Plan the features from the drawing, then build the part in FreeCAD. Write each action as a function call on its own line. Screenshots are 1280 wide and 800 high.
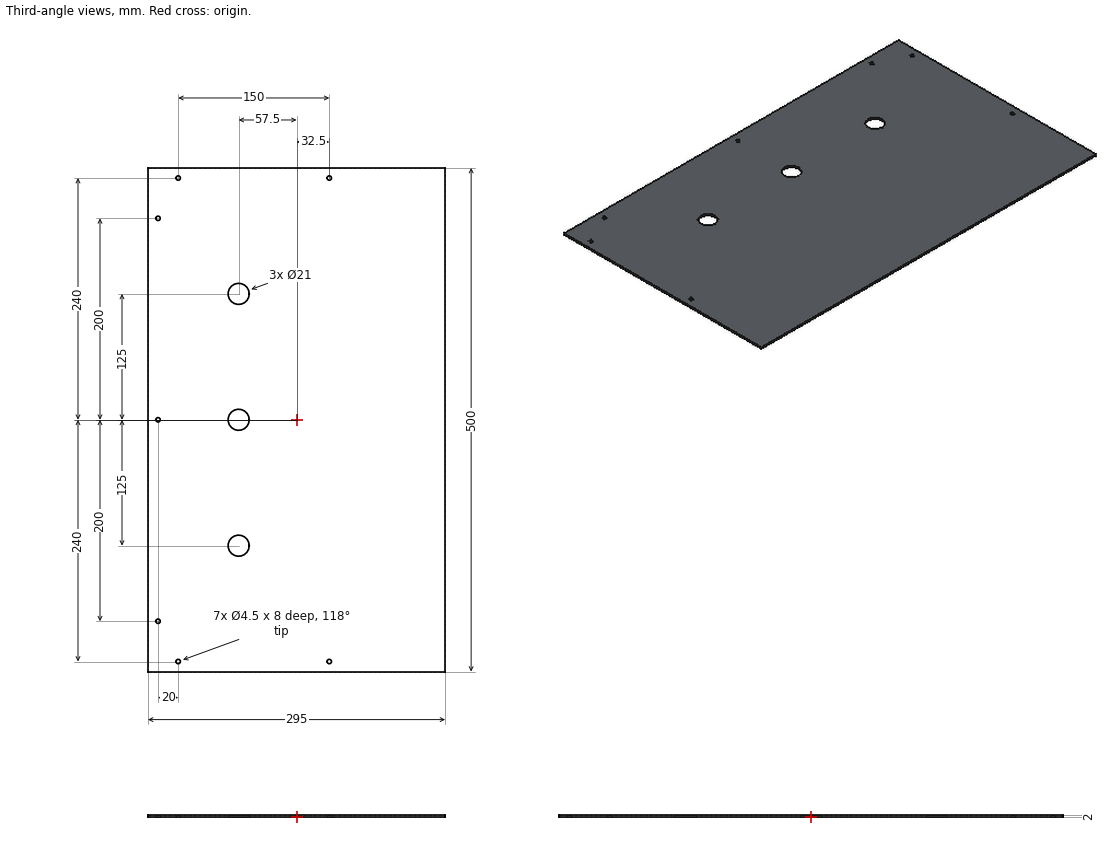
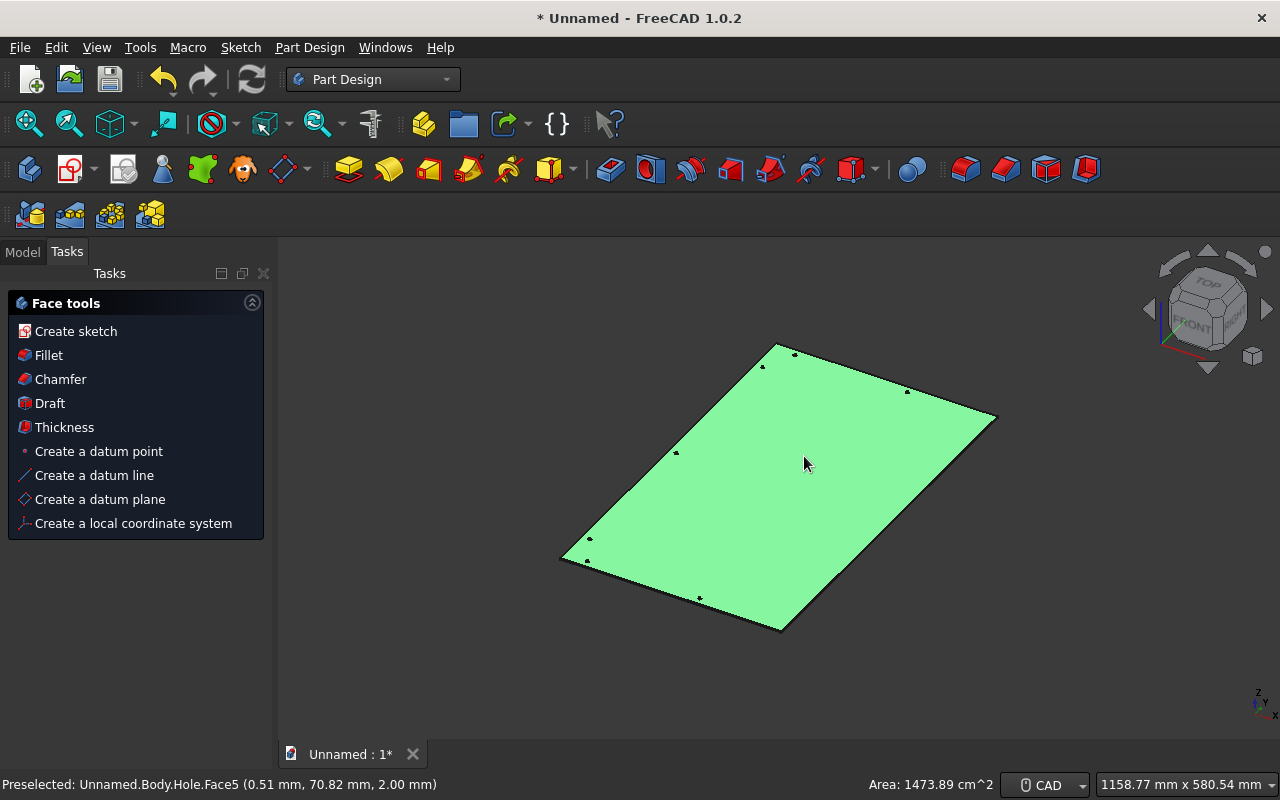
click(70, 170)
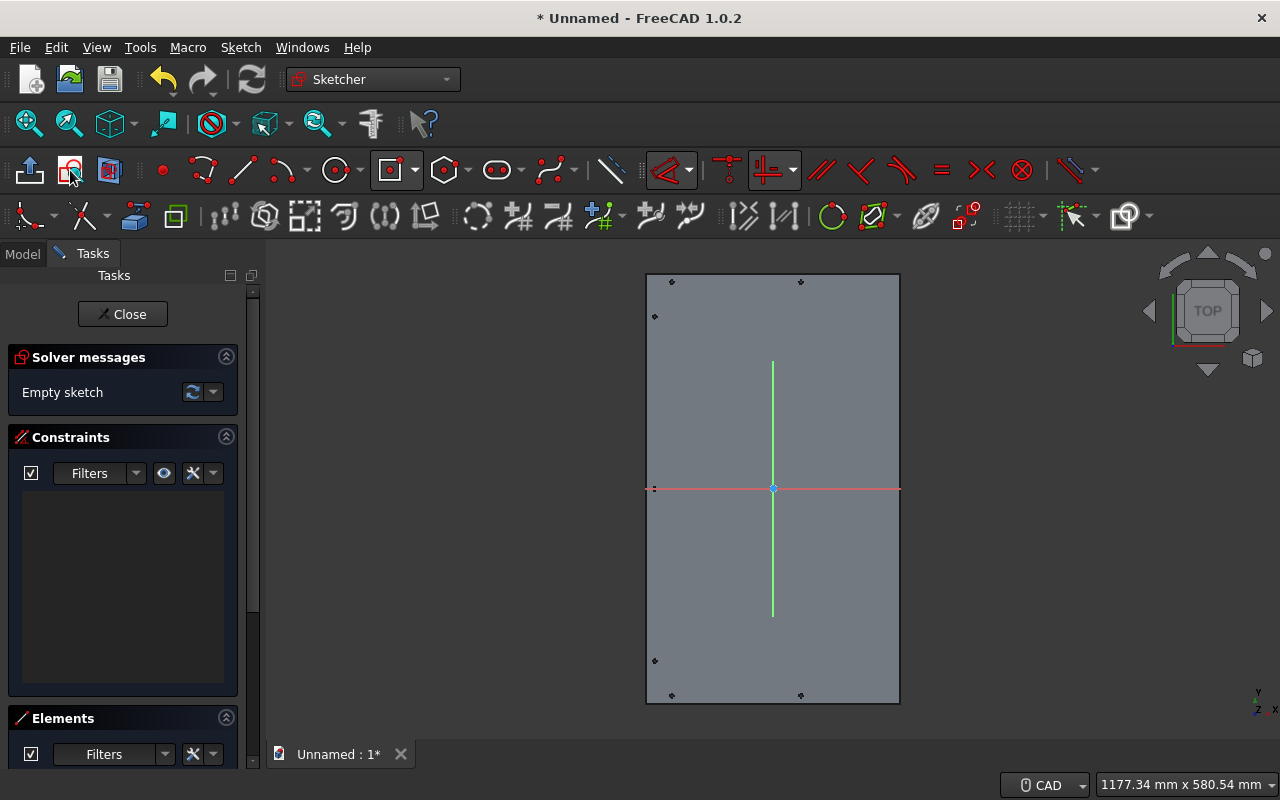
key(g)
key(c)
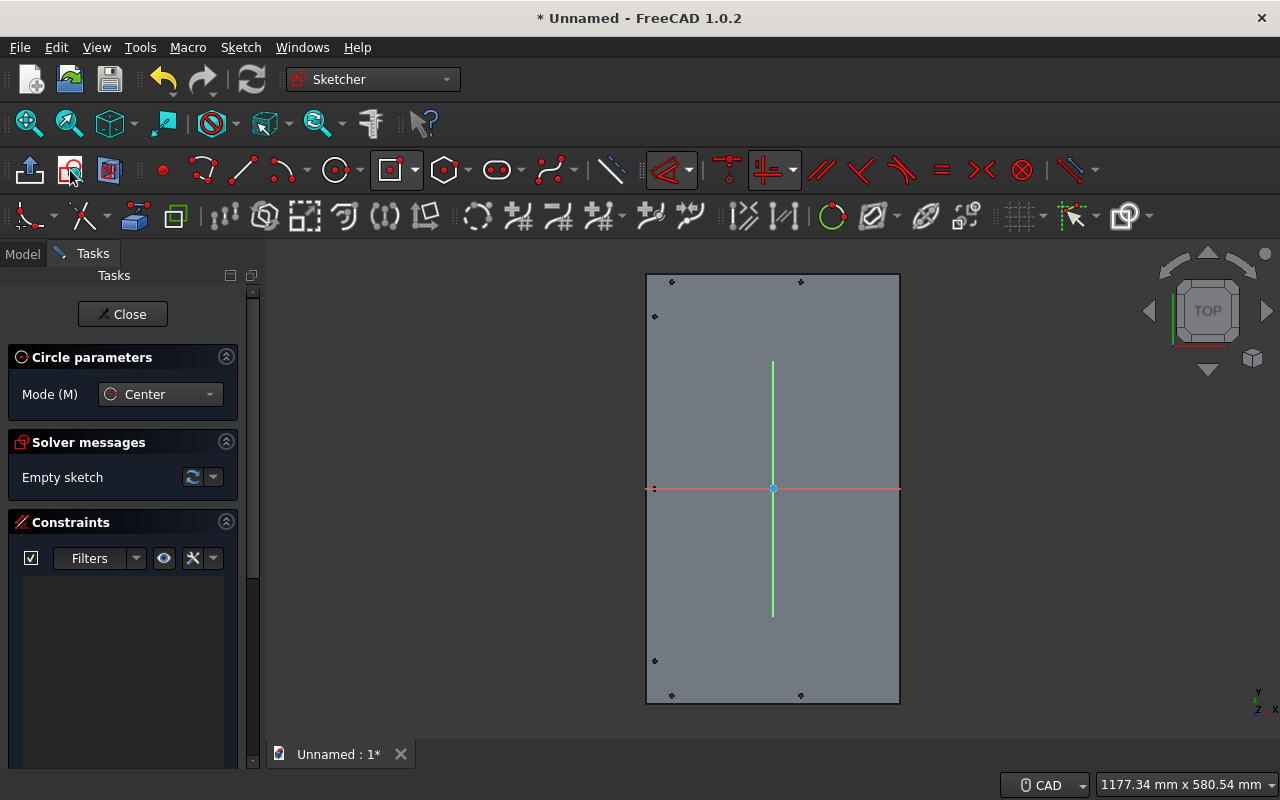
scroll(723, 381, up, 5)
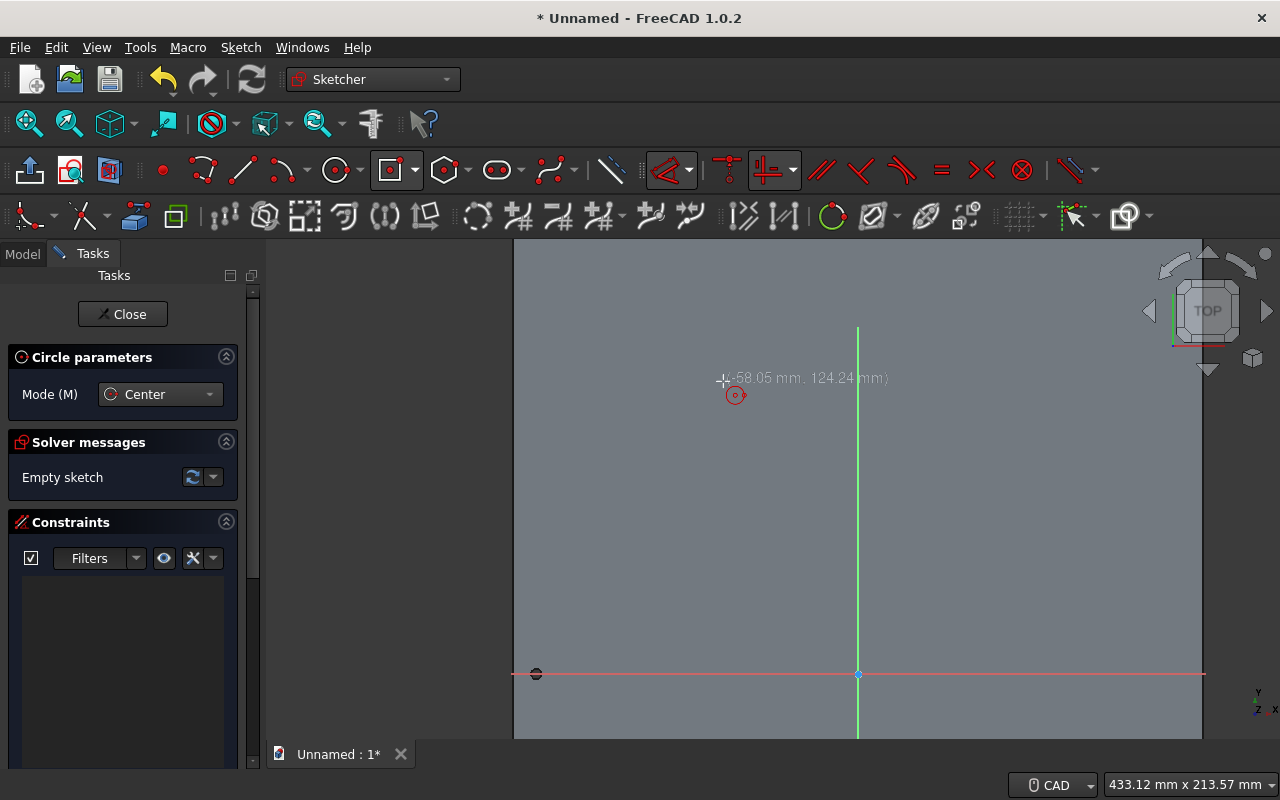
click(724, 381)
move(741, 364)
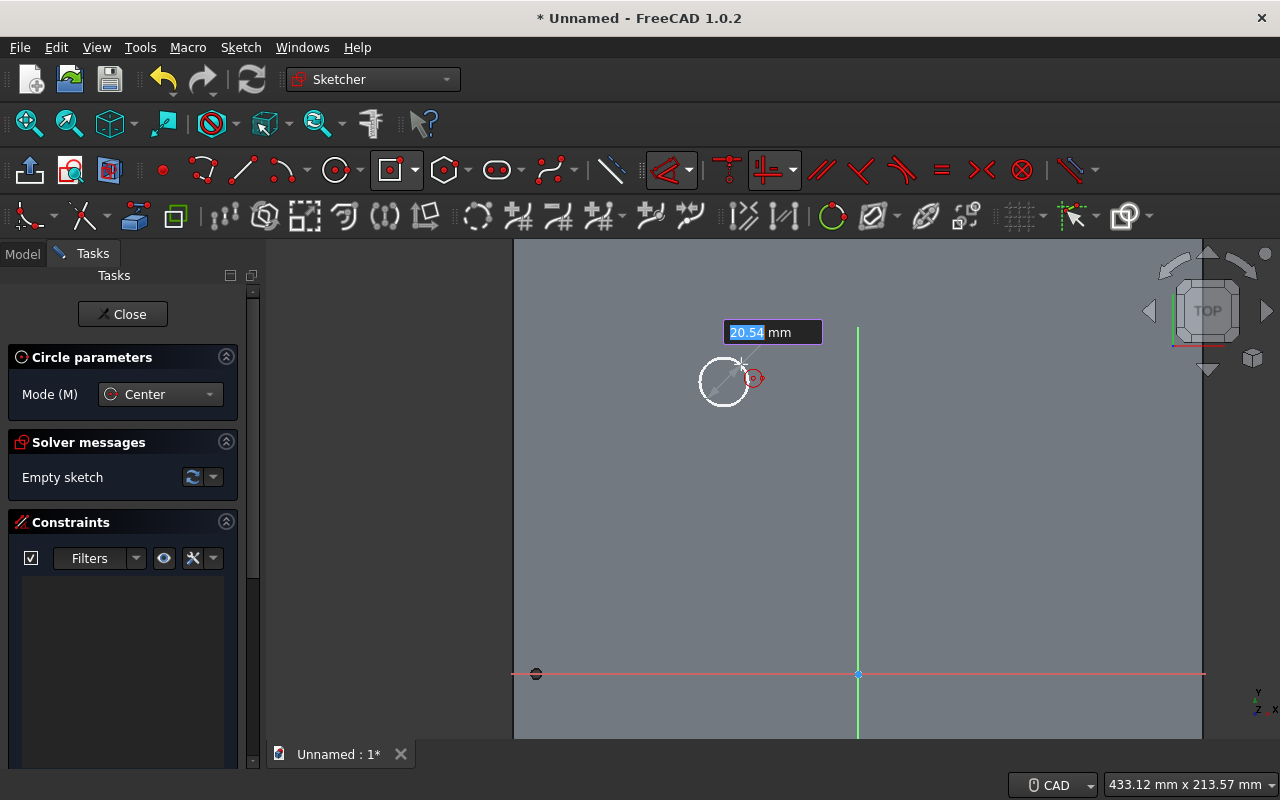
text(21)
key(Return)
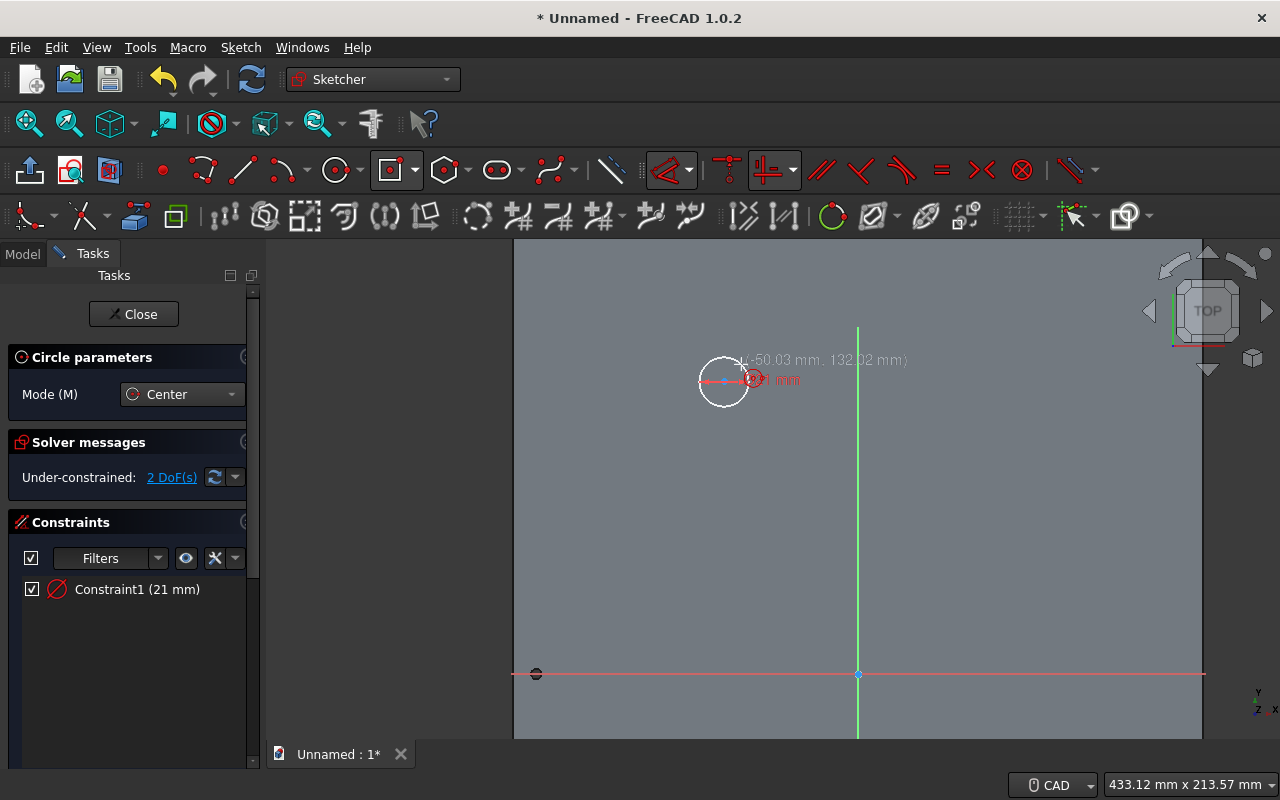
scroll(644, 338, down, 4)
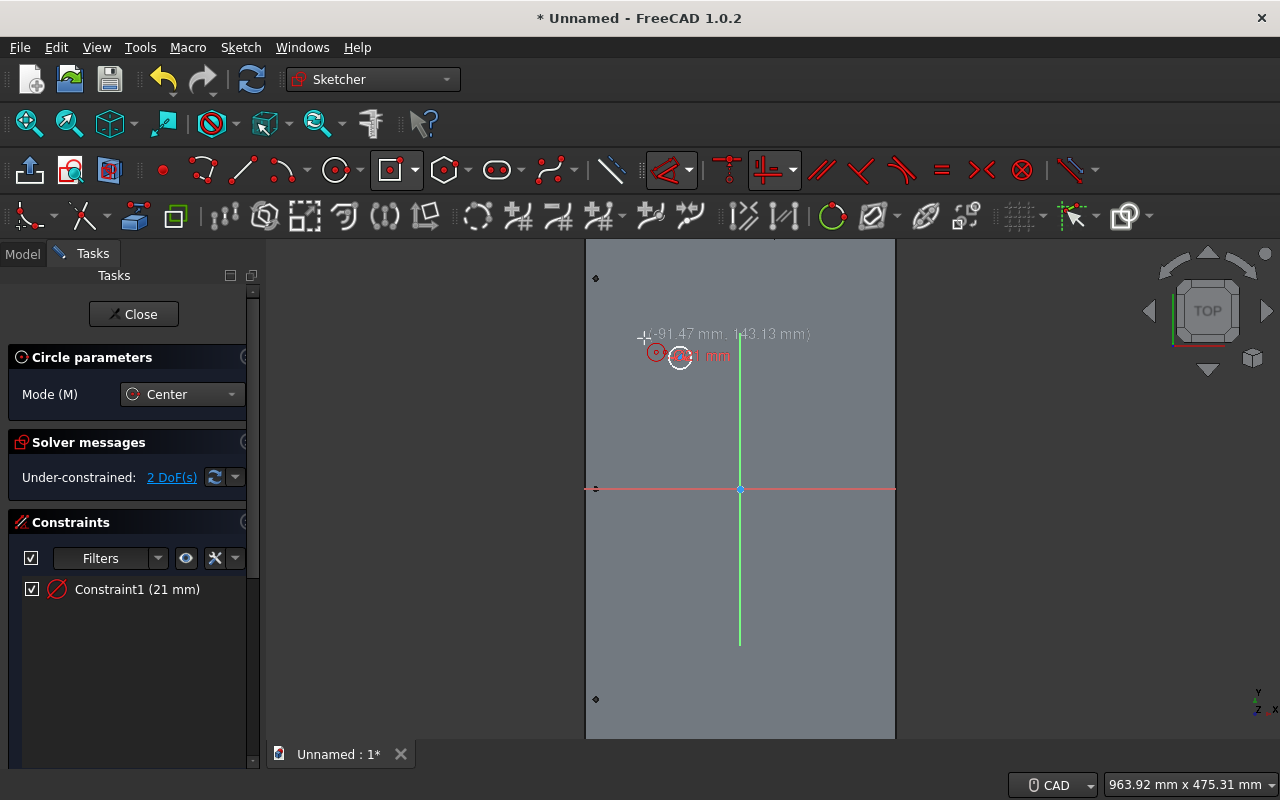
scroll(680, 621, up, 4)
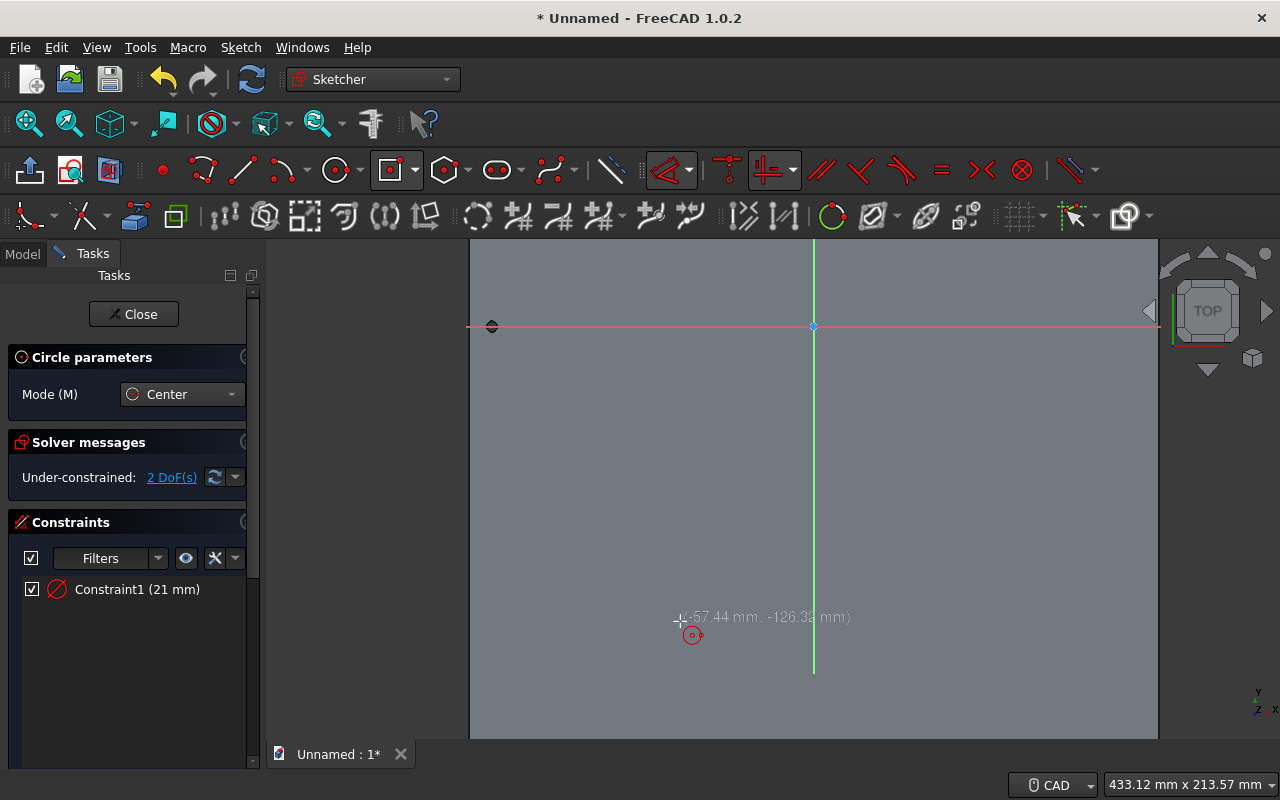
click(679, 619)
move(697, 602)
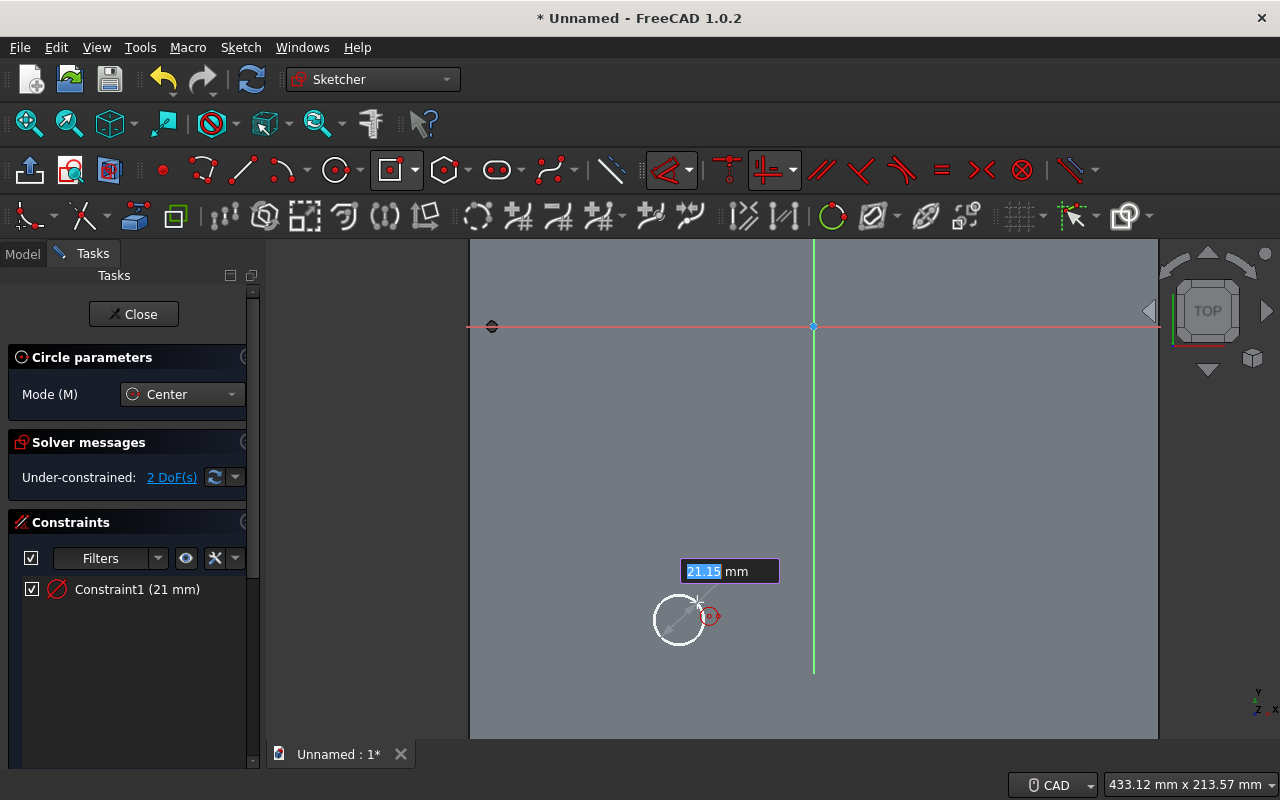
text(21)
key(Return)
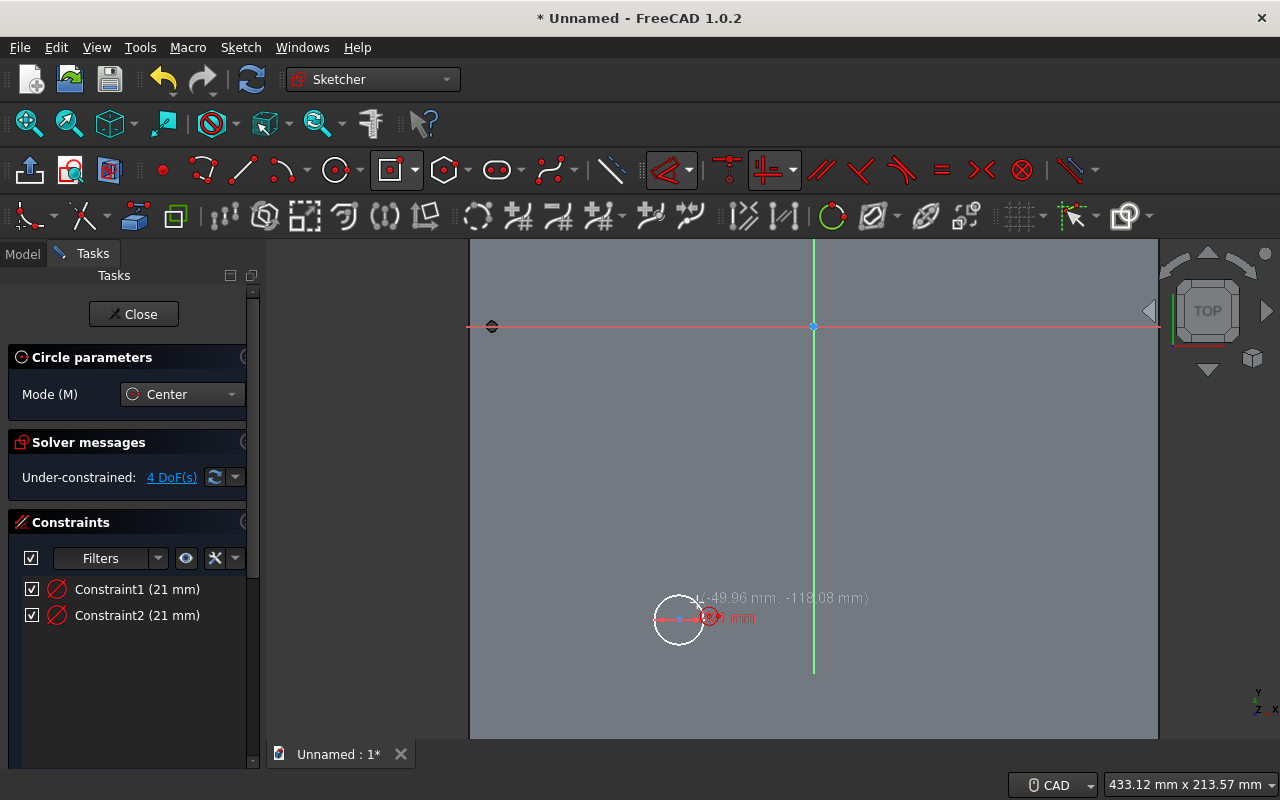
click(679, 327)
move(697, 309)